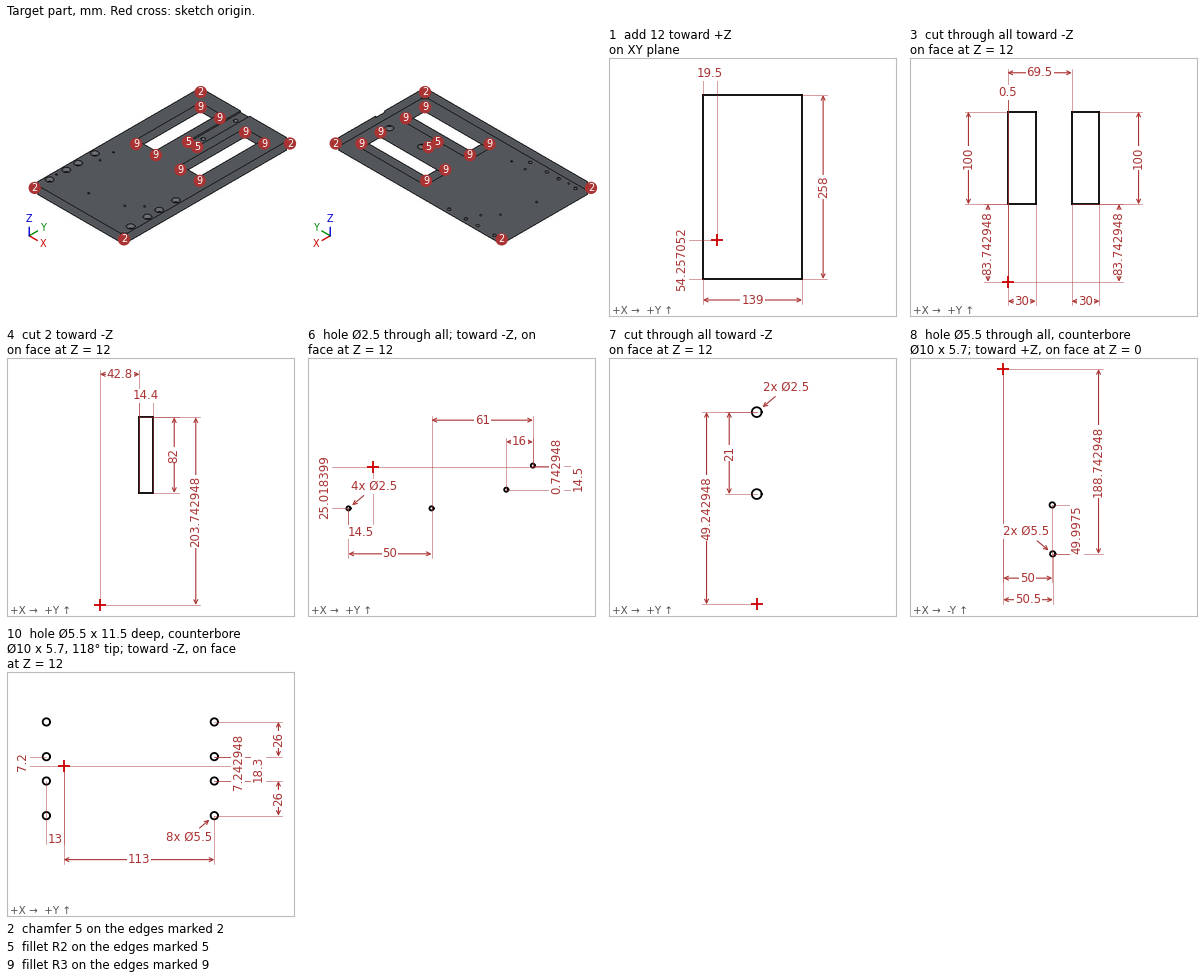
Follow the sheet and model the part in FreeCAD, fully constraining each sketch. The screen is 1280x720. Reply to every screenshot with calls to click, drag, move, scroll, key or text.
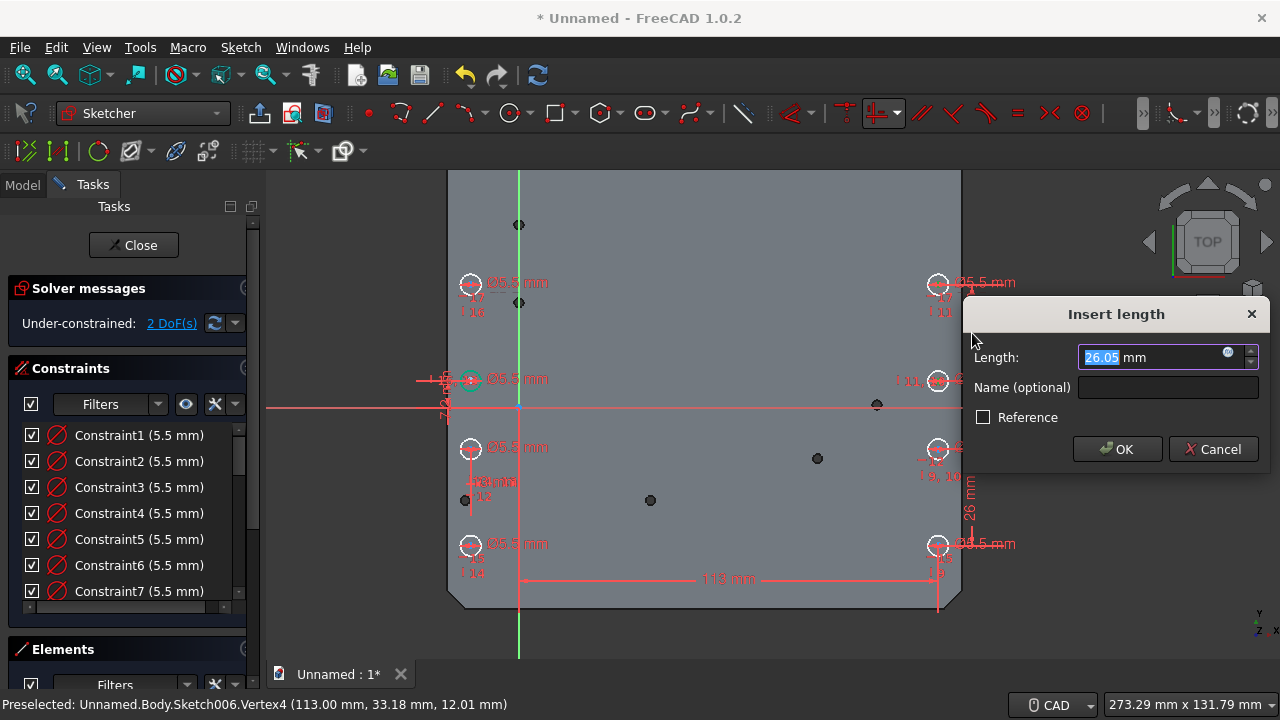
text(26)
key(Return)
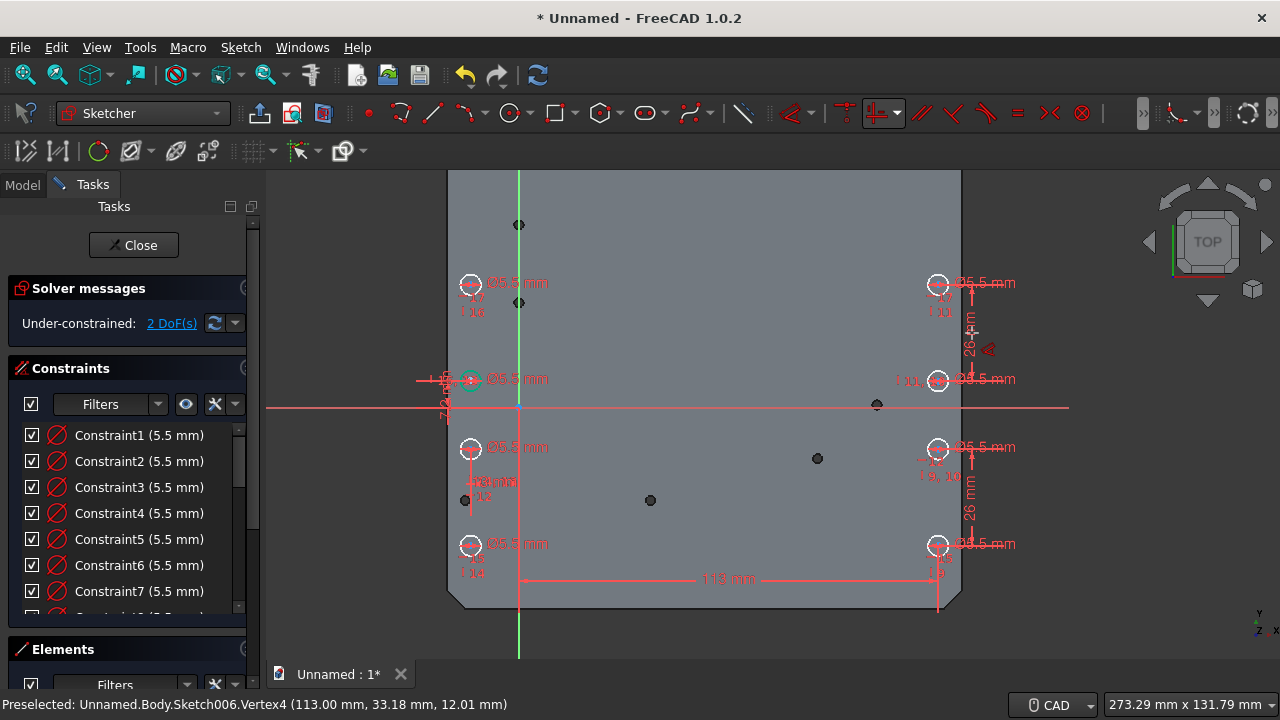
click(938, 449)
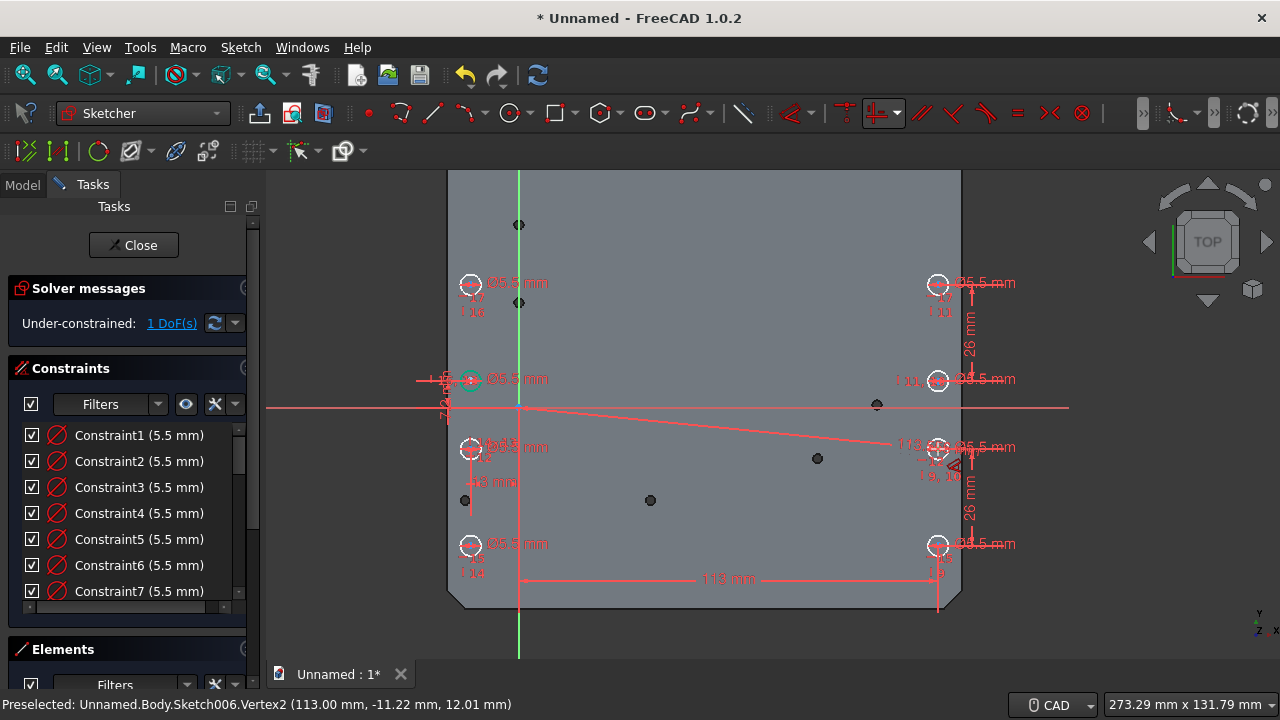
click(938, 381)
click(972, 431)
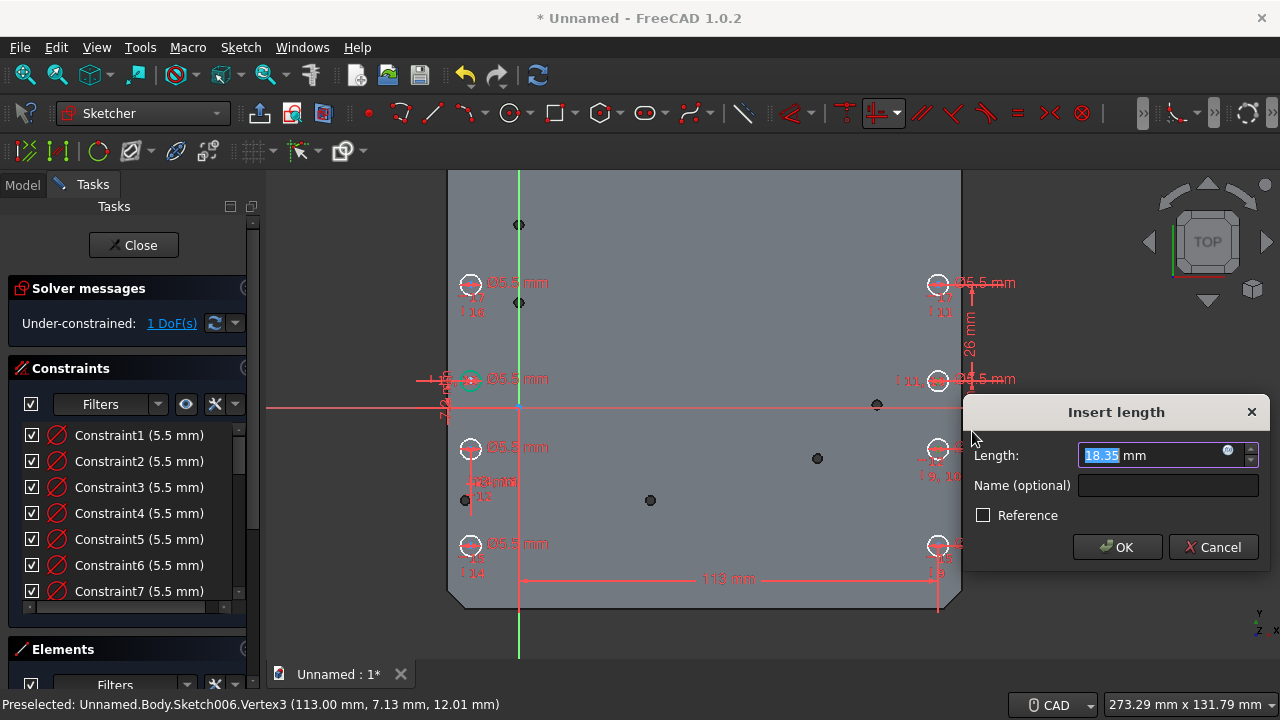
text(18.3)
key(Return)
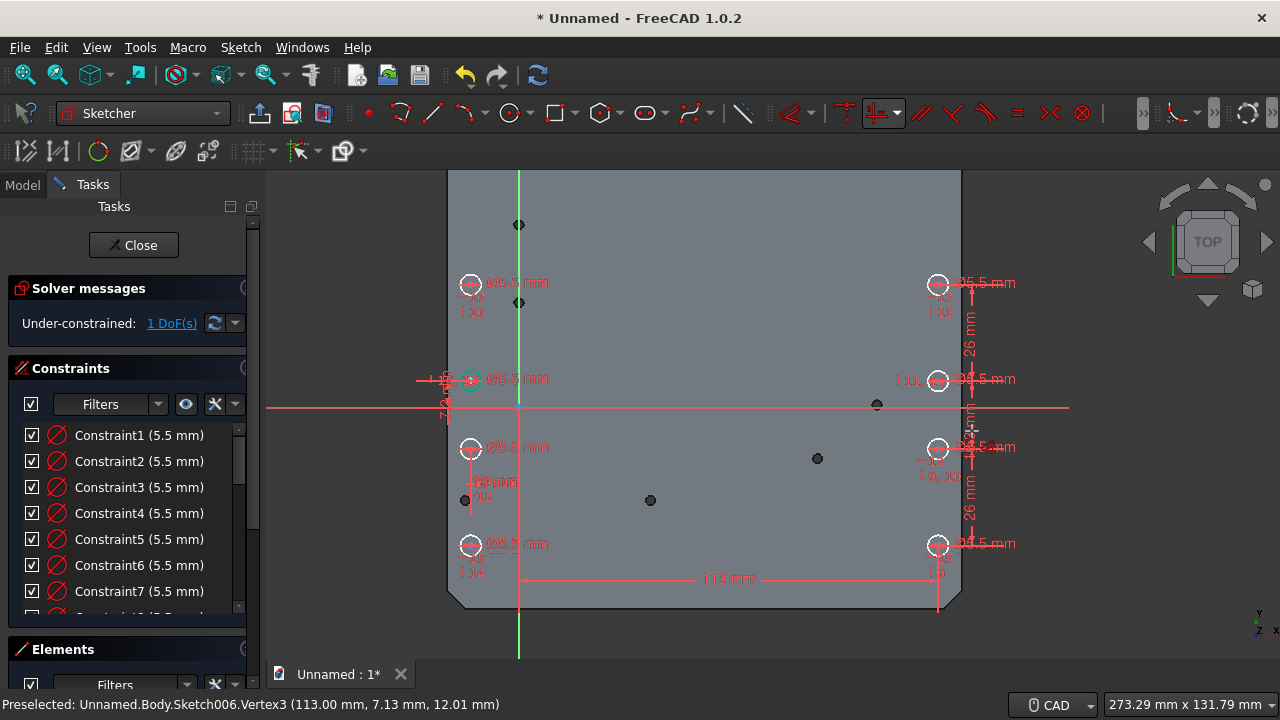
scroll(938, 381, up, 2)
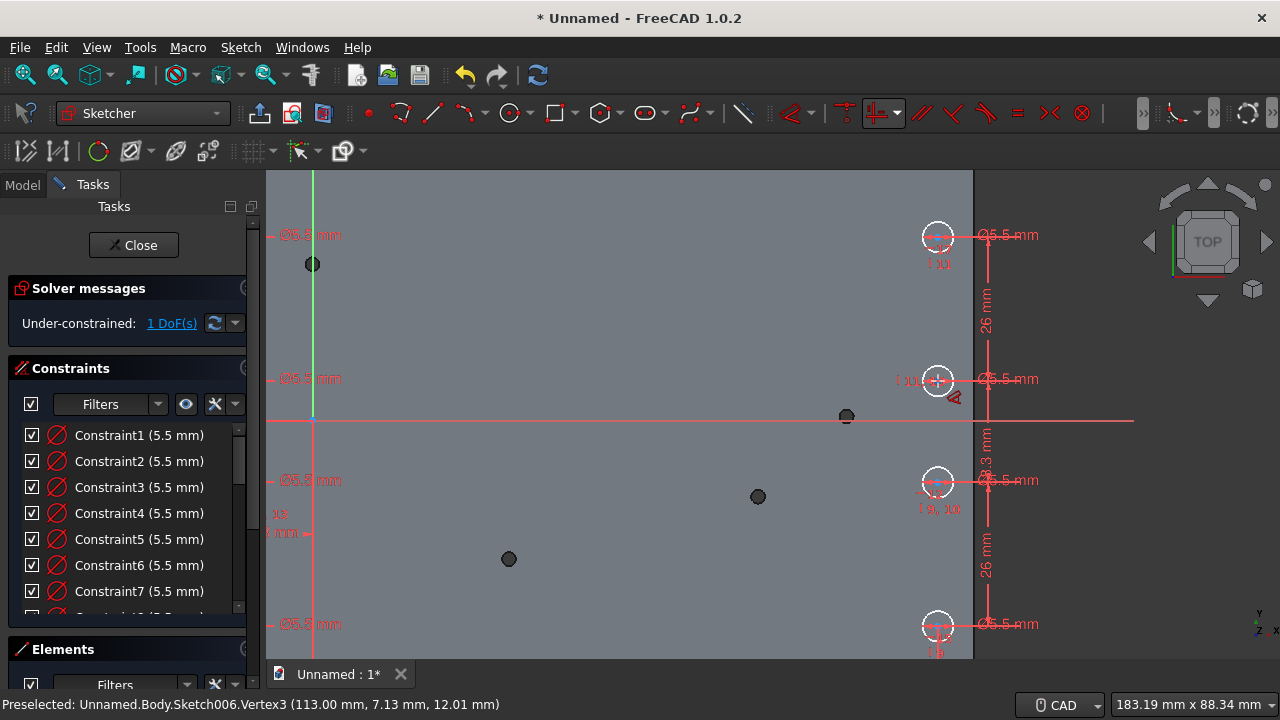
click(938, 381)
click(972, 401)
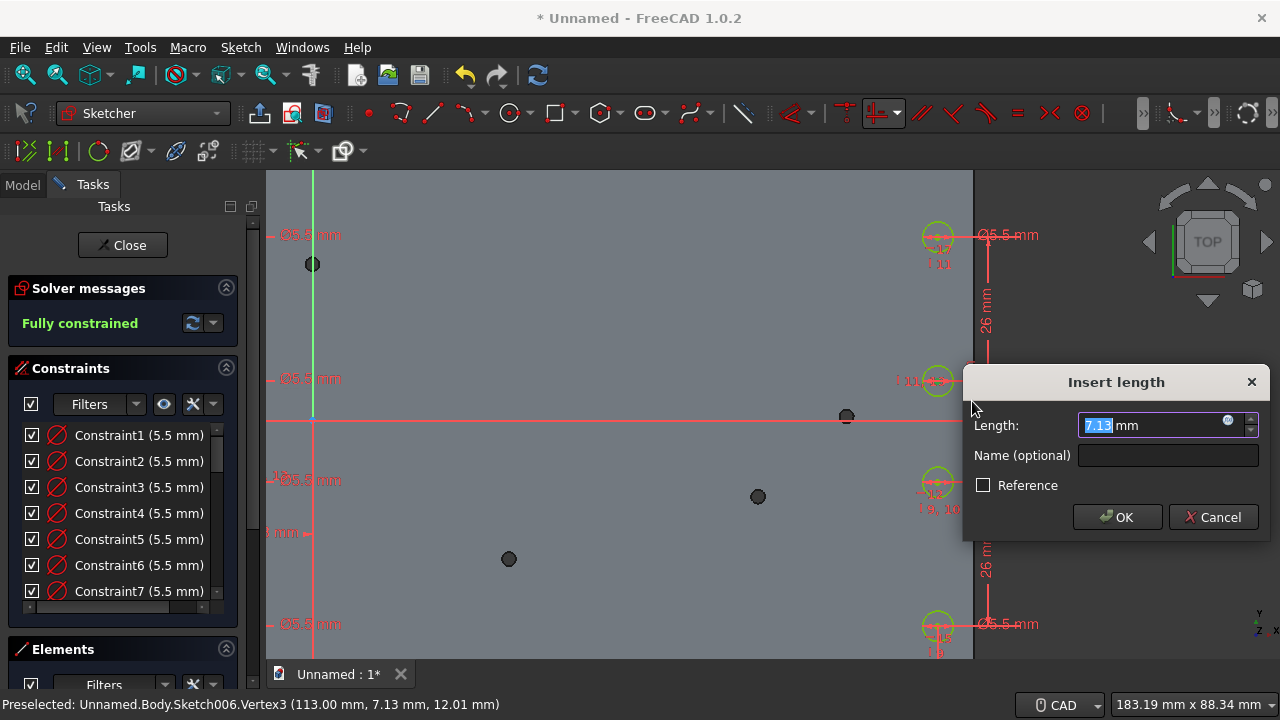
text(7.242948)
key(Return)
key(Escape)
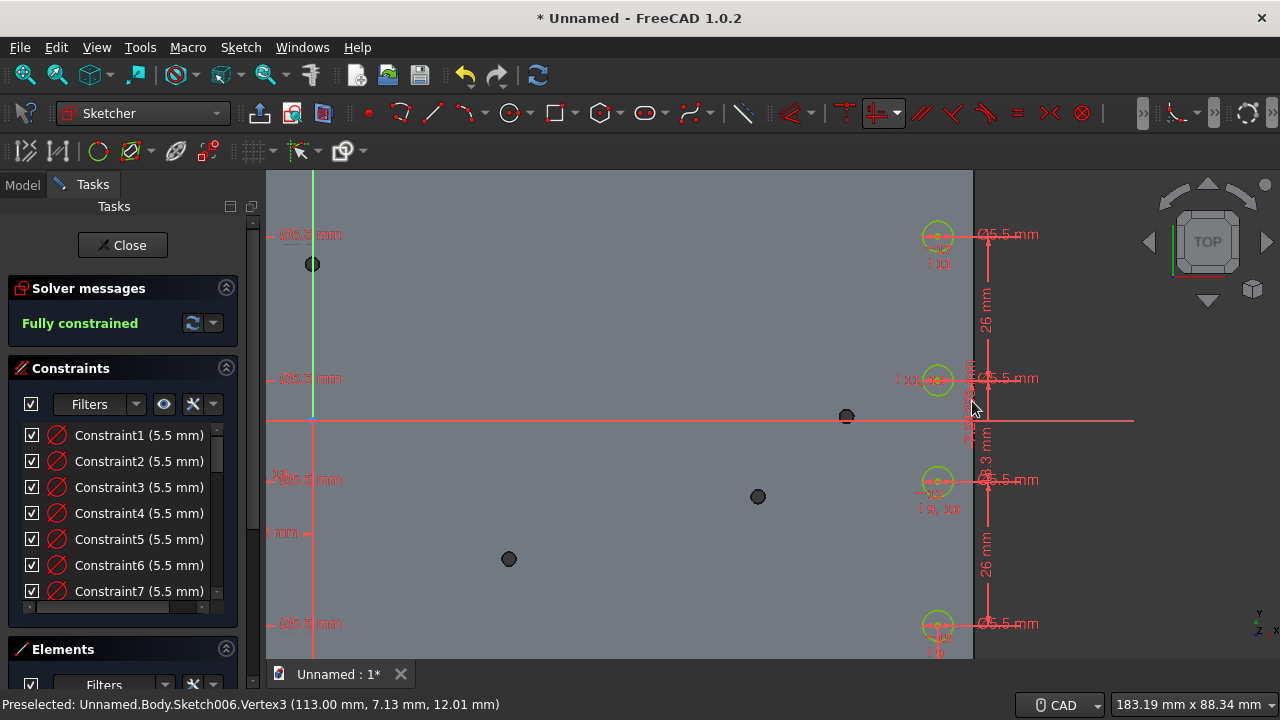
click(123, 245)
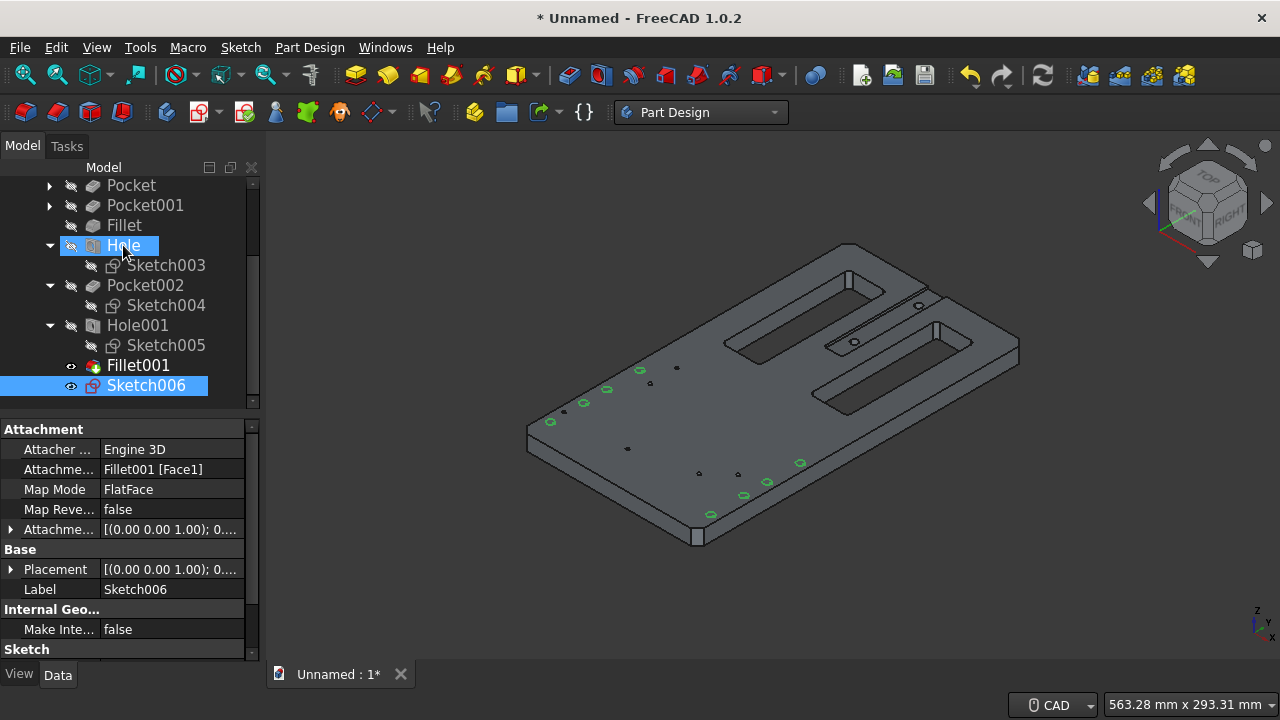
click(602, 76)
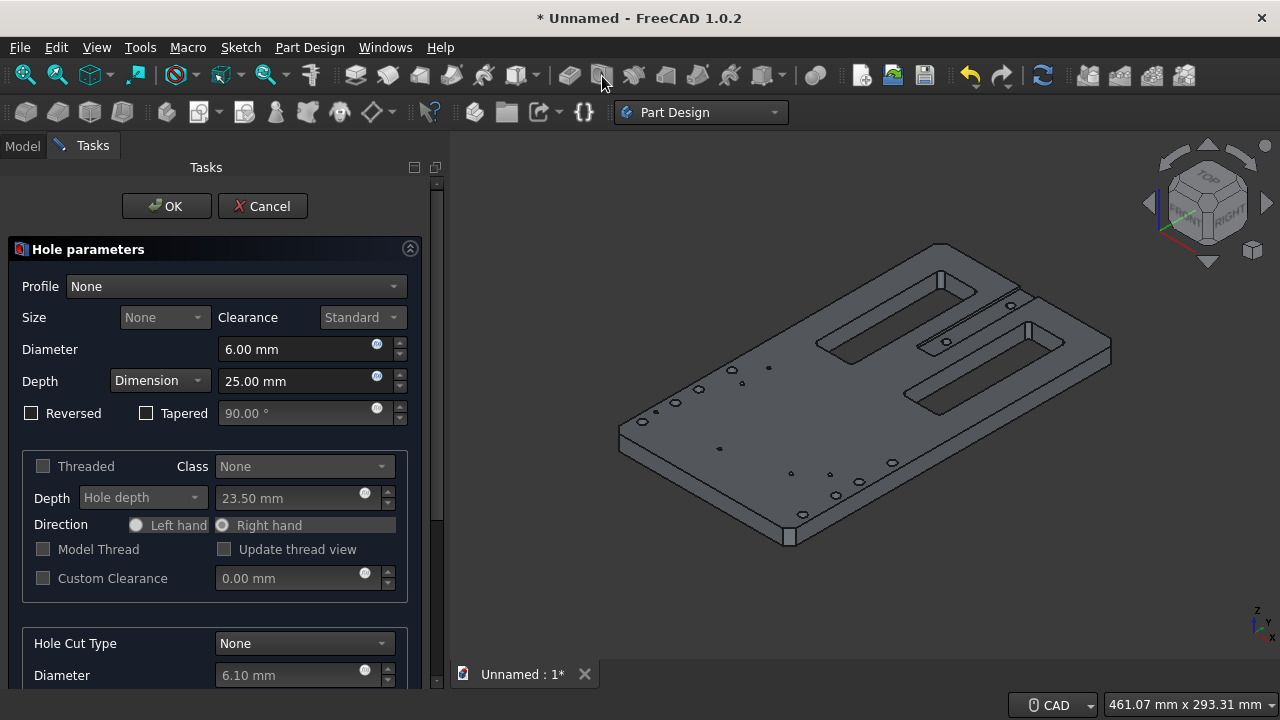
triple_click(305, 349)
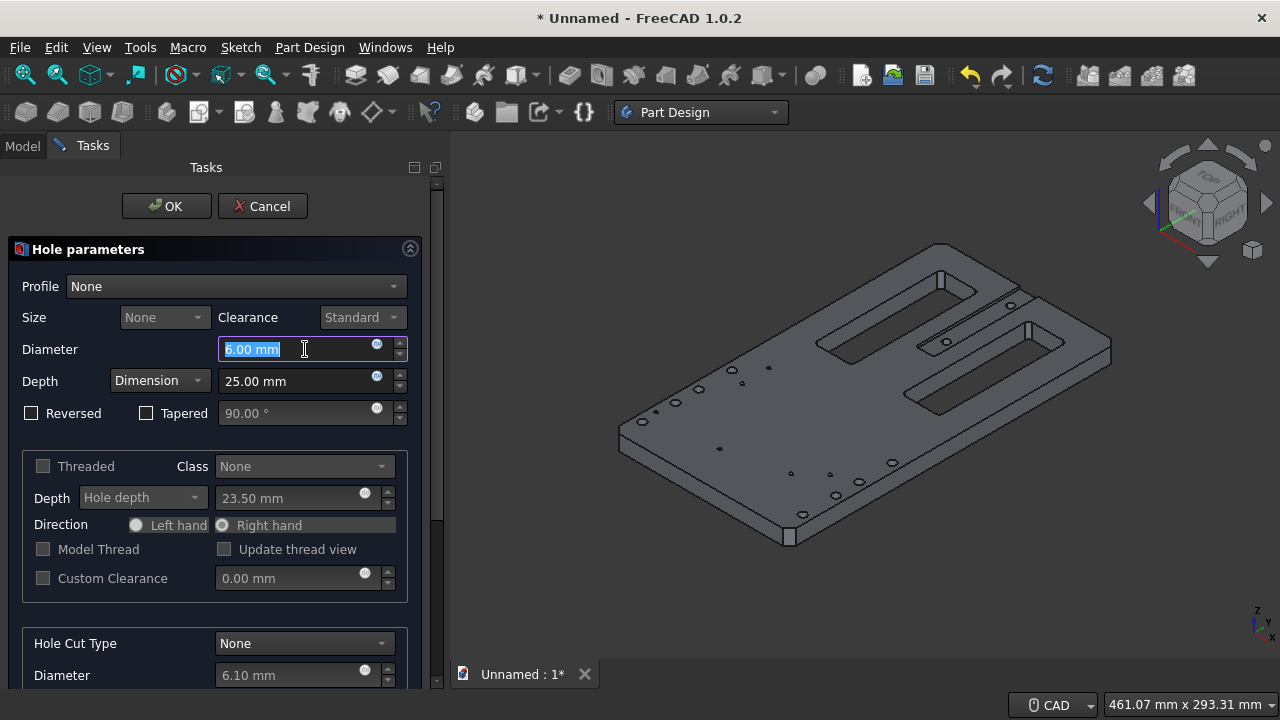
text(5.5)
key(Tab)